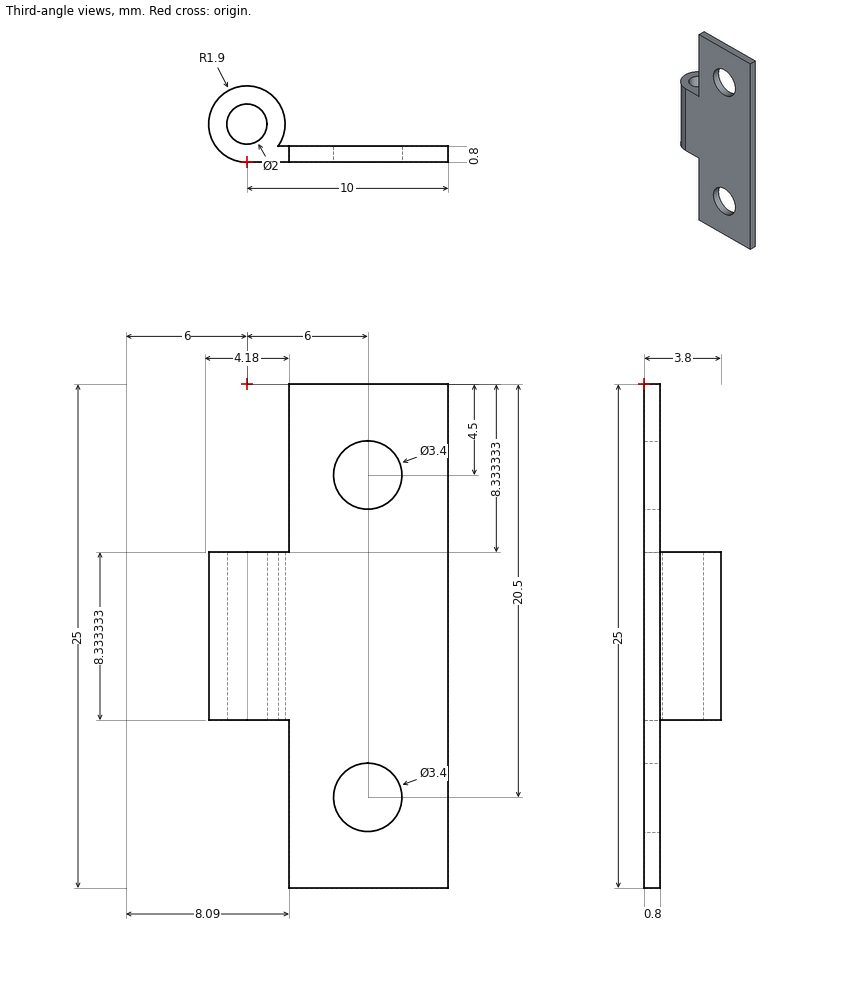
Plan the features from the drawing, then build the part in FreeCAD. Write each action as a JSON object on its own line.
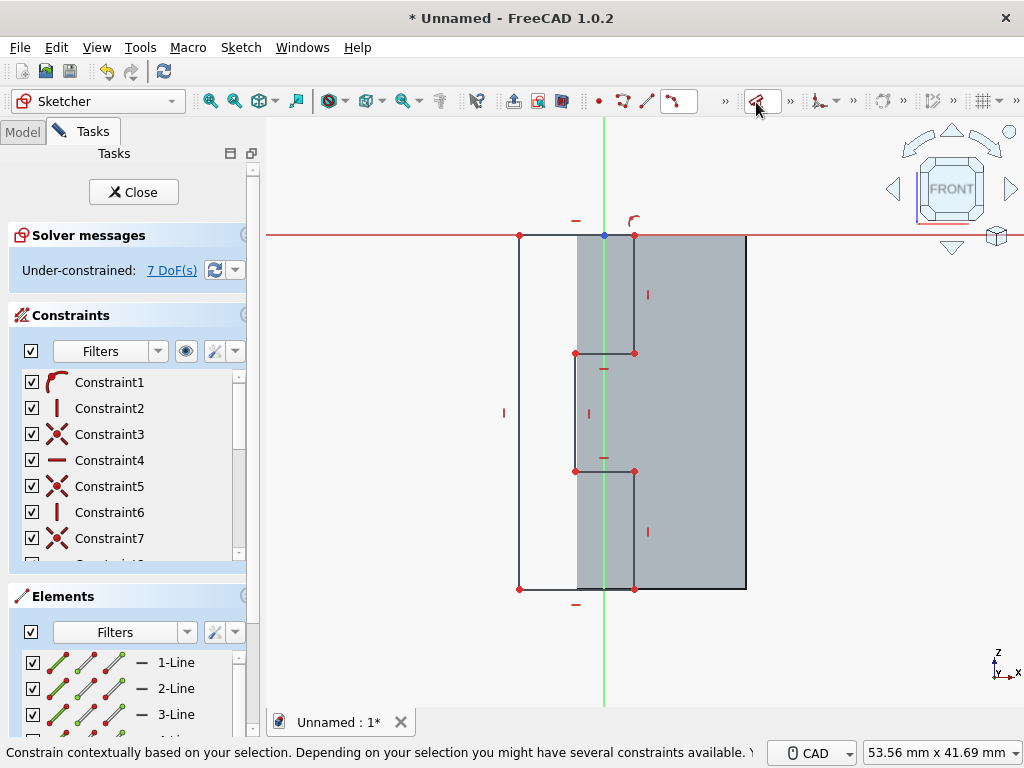
{"action": "left_click", "coordinate": [519, 484]}
{"action": "left_click", "coordinate": [485, 413]}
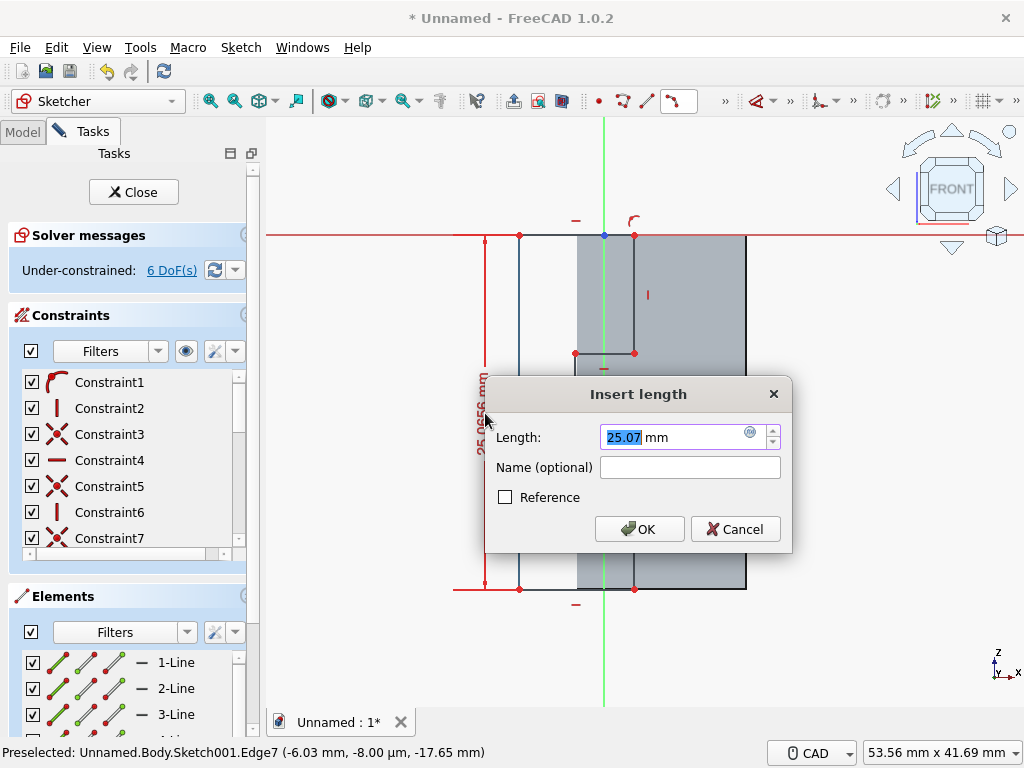
{"action": "type", "text": "25"}
{"action": "key", "text": "Return"}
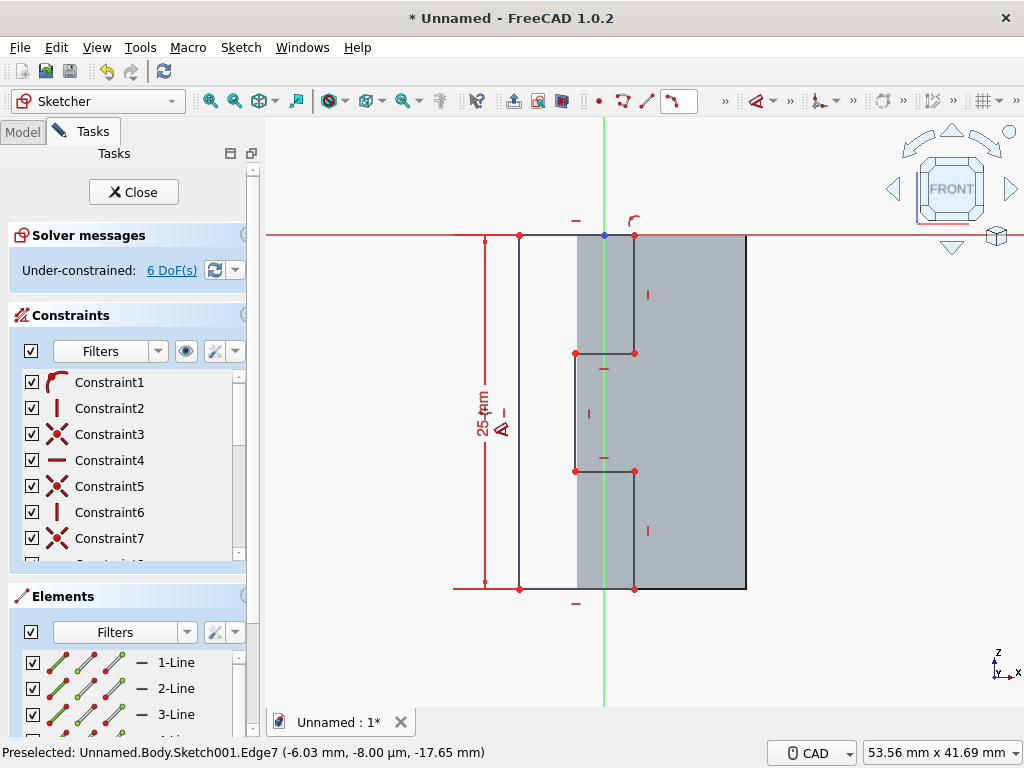
{"action": "left_click", "coordinate": [519, 589]}
{"action": "left_click", "coordinate": [562, 623]}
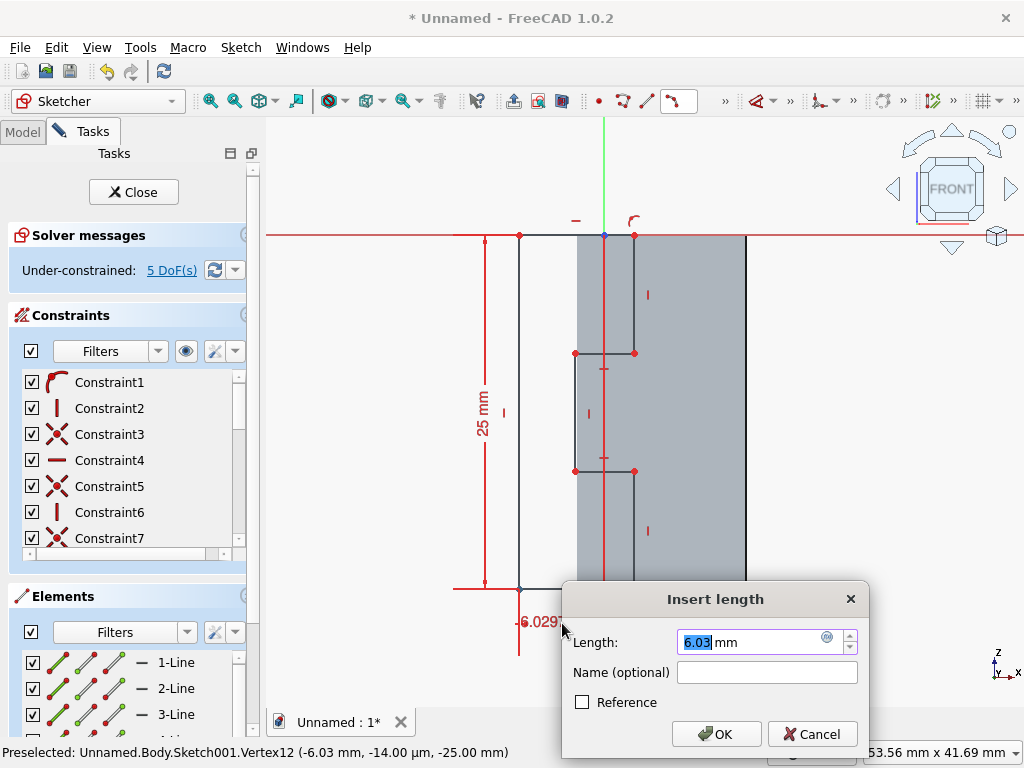
{"action": "type", "text": "6"}
{"action": "key", "text": "Return"}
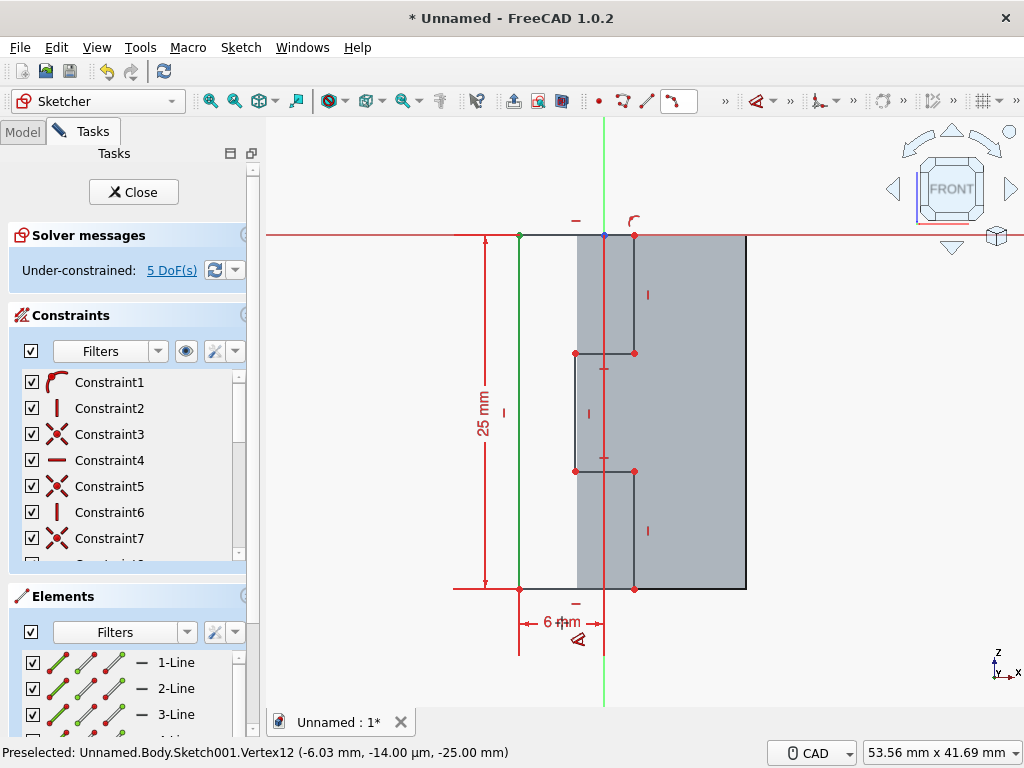
{"action": "left_click", "coordinate": [616, 354]}
{"action": "left_click", "coordinate": [591, 320]}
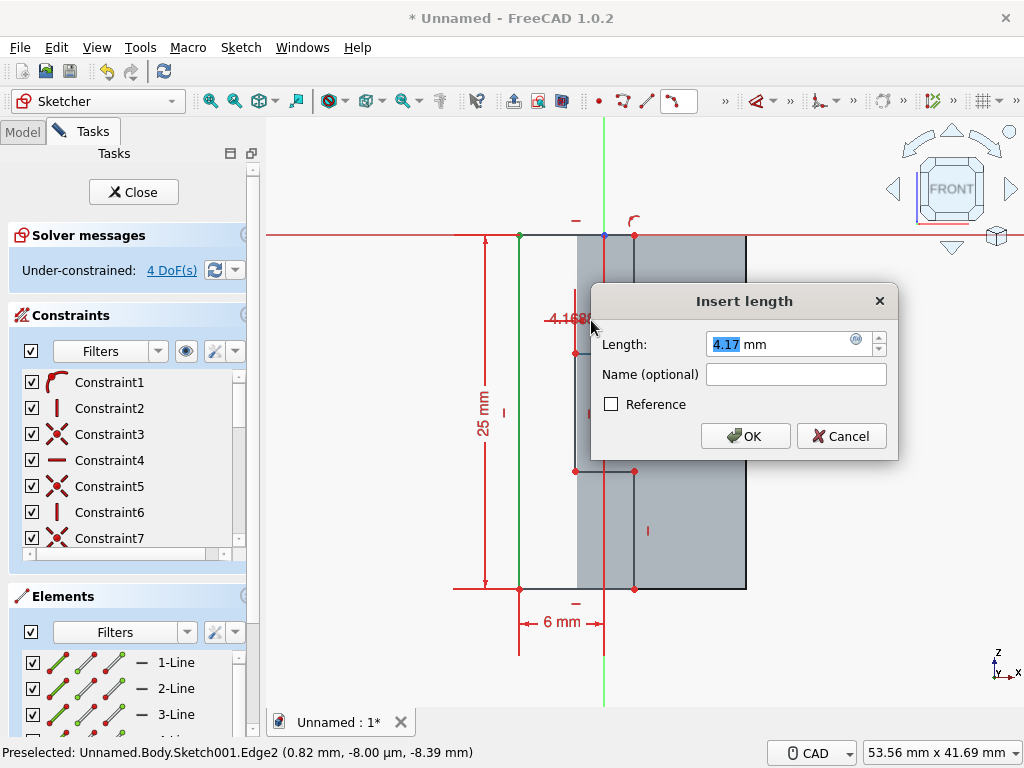
{"action": "type", "text": "4.18"}
{"action": "key", "text": "Return"}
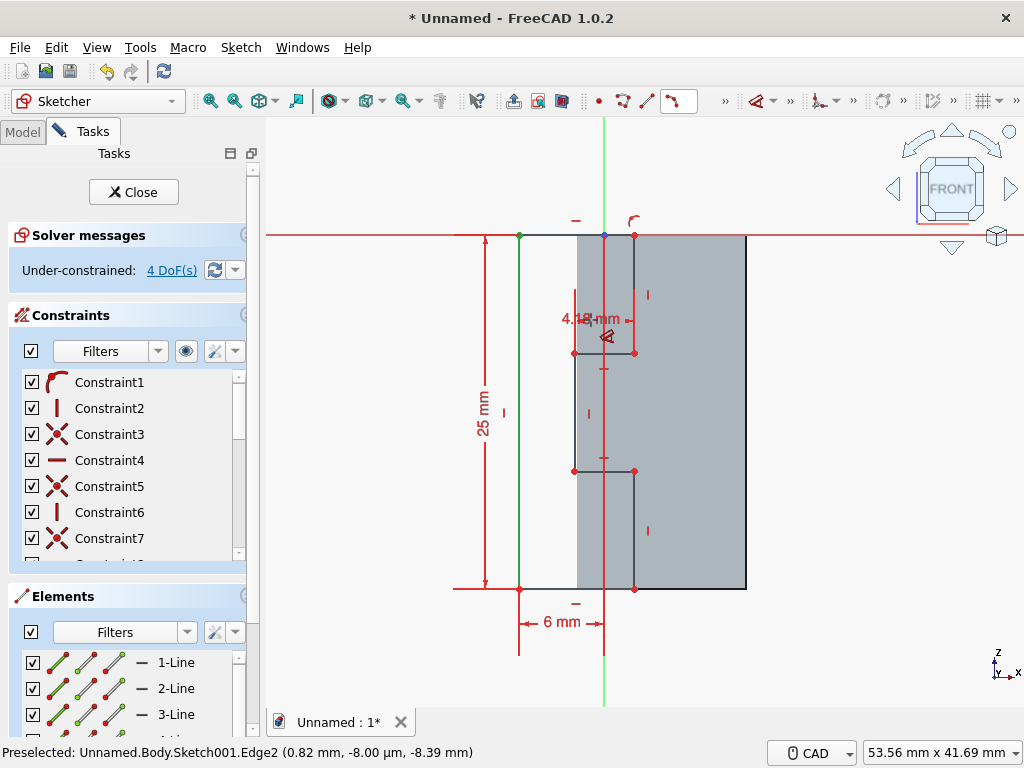
{"action": "left_click", "coordinate": [593, 472]}
{"action": "left_click", "coordinate": [591, 506]}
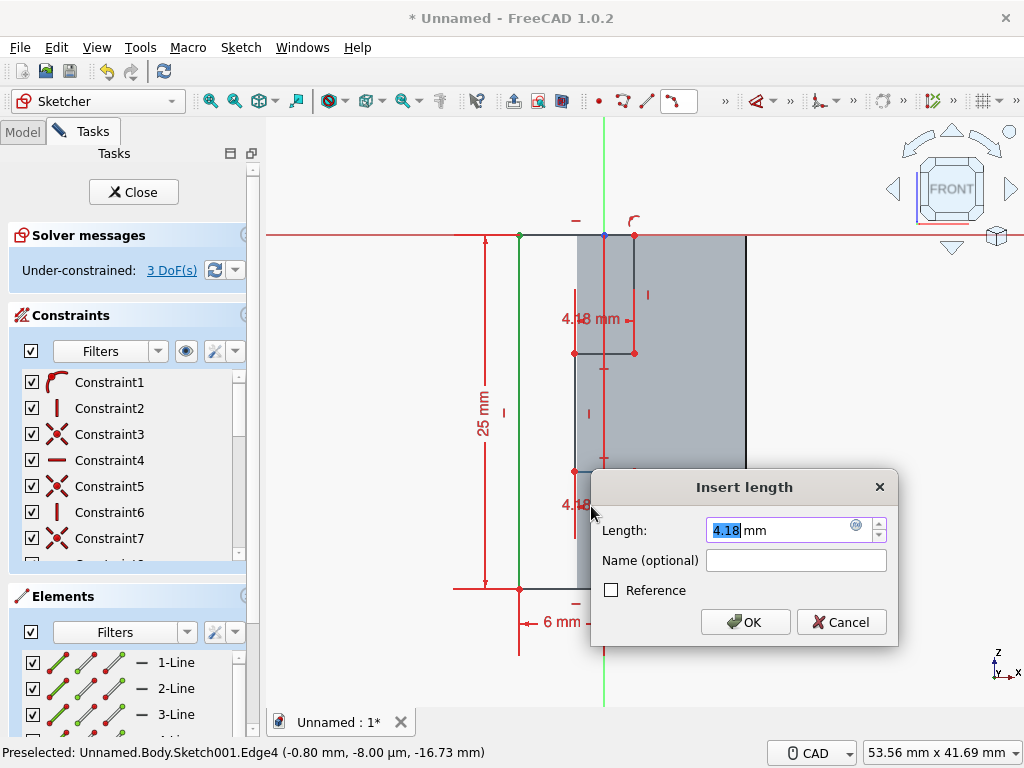
{"action": "type", "text": "4.18"}
{"action": "key", "text": "Return"}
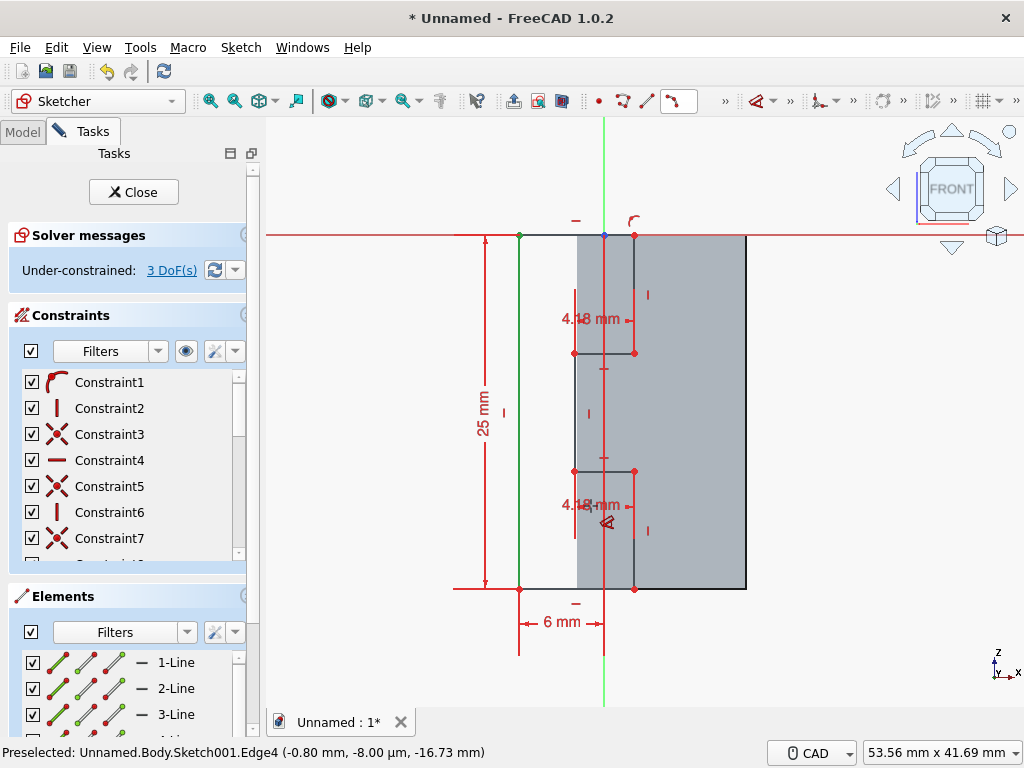
{"action": "left_click", "coordinate": [554, 589]}
{"action": "left_click", "coordinate": [577, 555]}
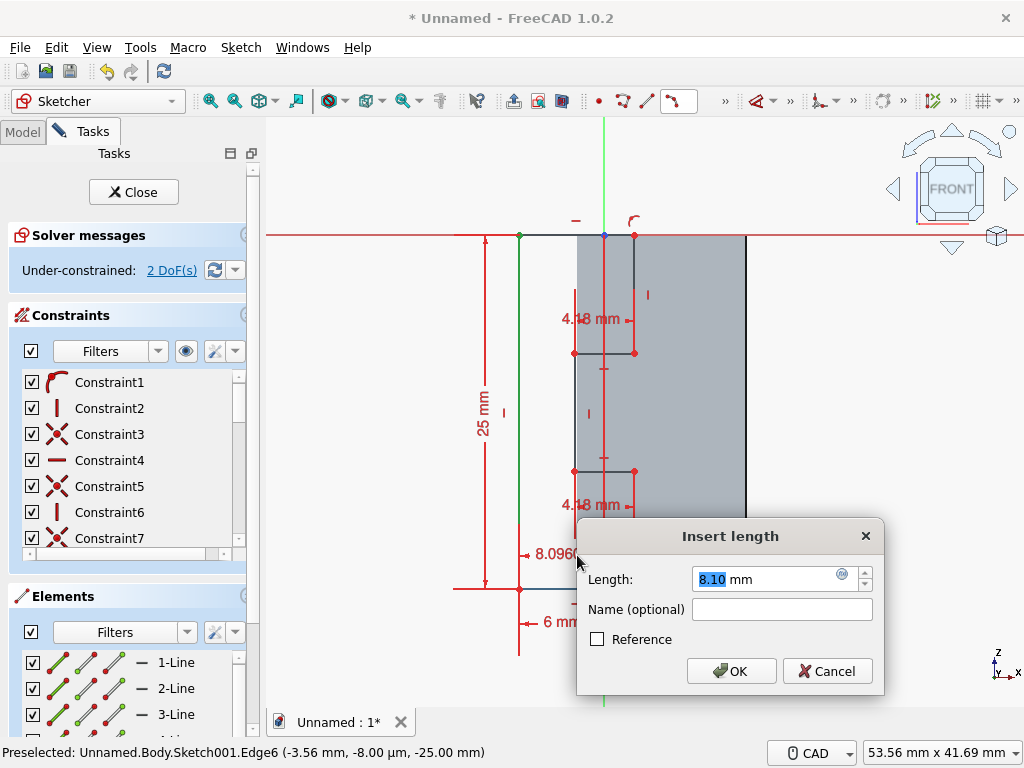
{"action": "type", "text": "8.09"}
{"action": "key", "text": "Return"}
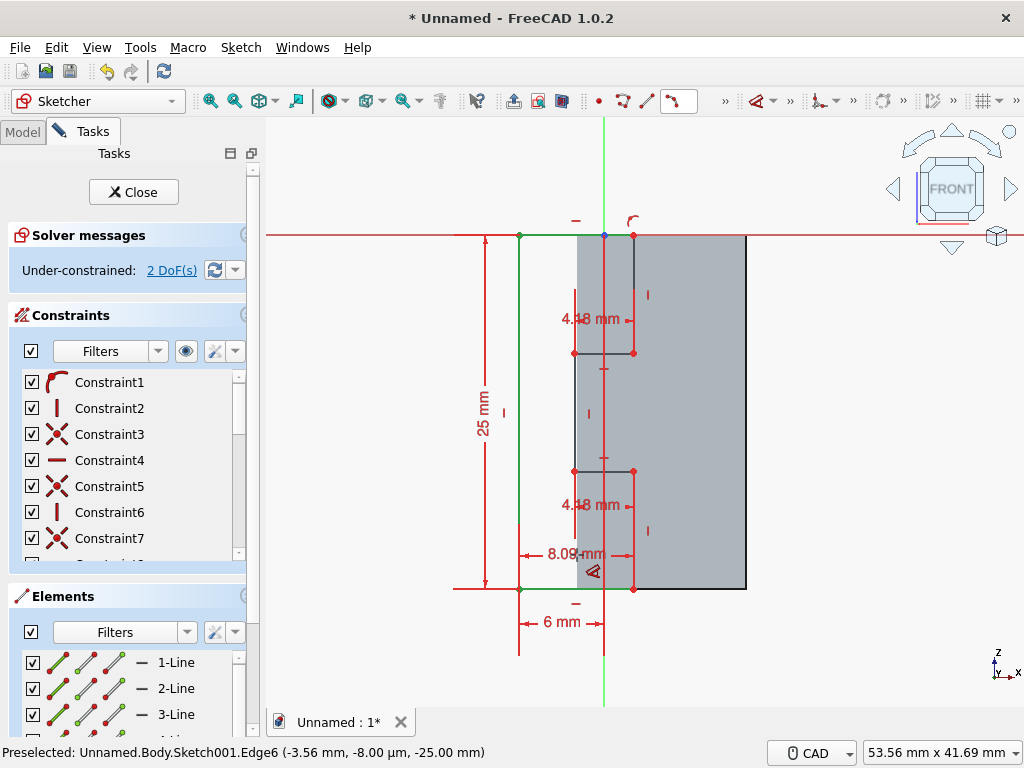
{"action": "left_click", "coordinate": [634, 271]}
{"action": "left_click", "coordinate": [668, 295]}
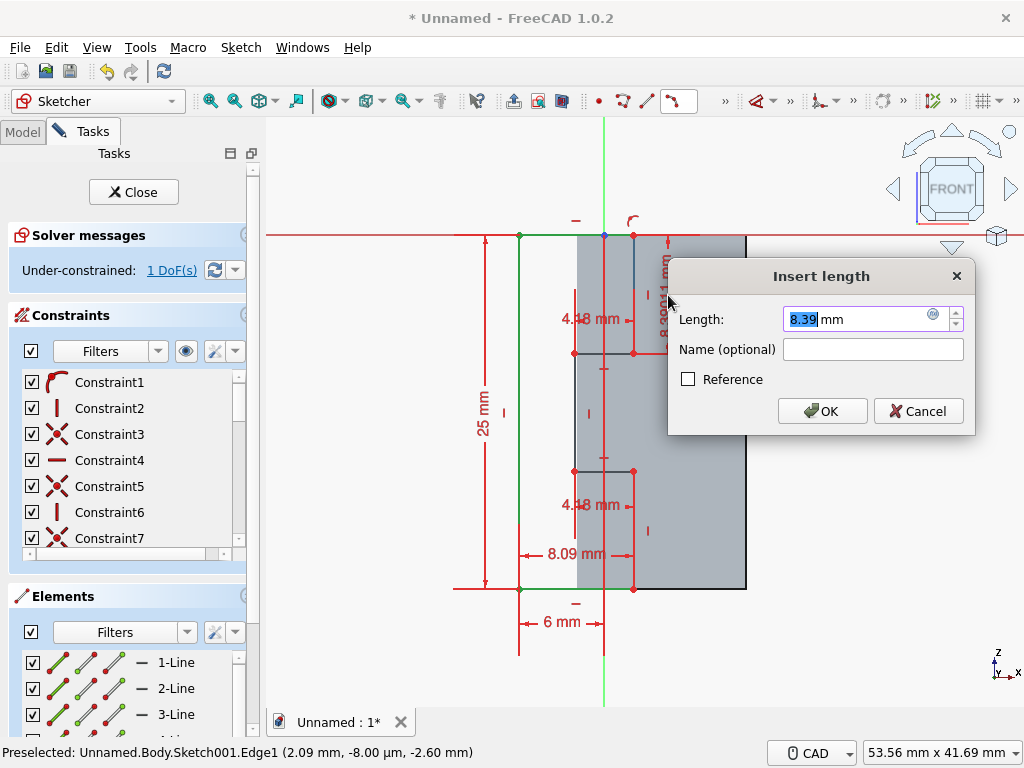
{"action": "type", "text": "8.333333"}
{"action": "key", "text": "Return"}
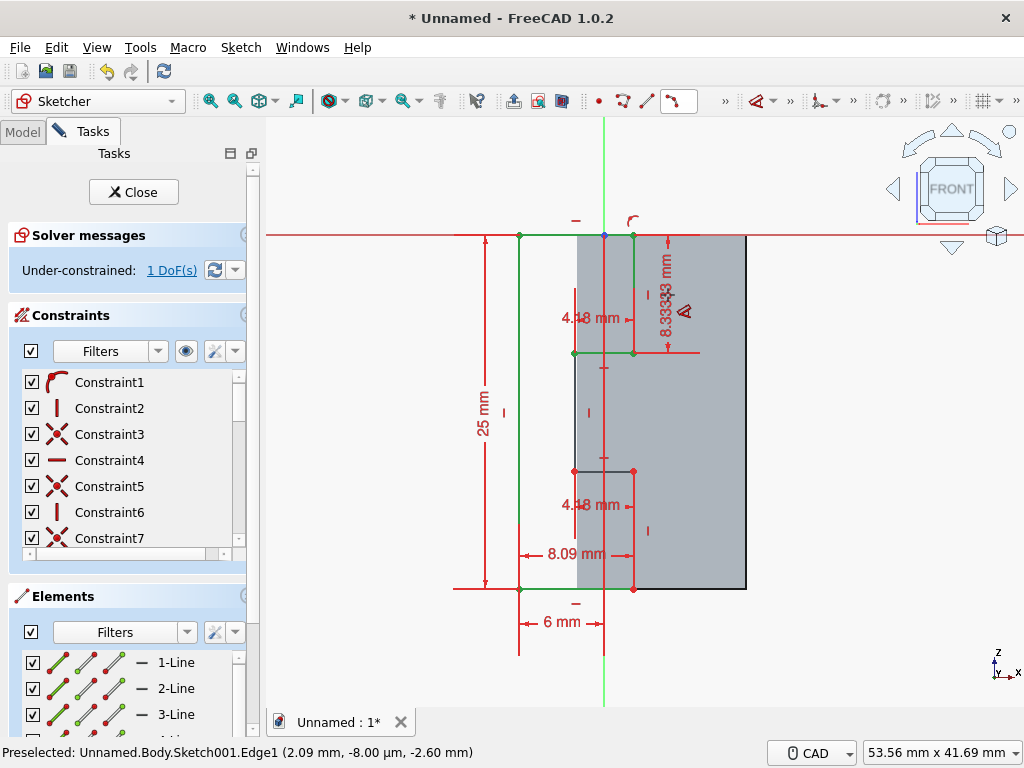
{"action": "left_click", "coordinate": [575, 389]}
{"action": "left_click", "coordinate": [541, 385]}